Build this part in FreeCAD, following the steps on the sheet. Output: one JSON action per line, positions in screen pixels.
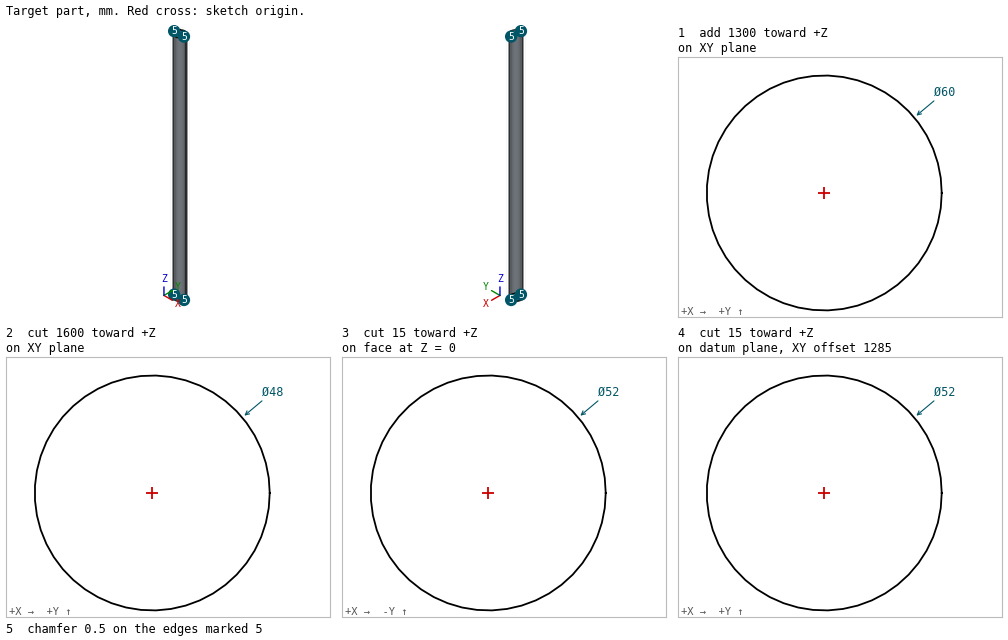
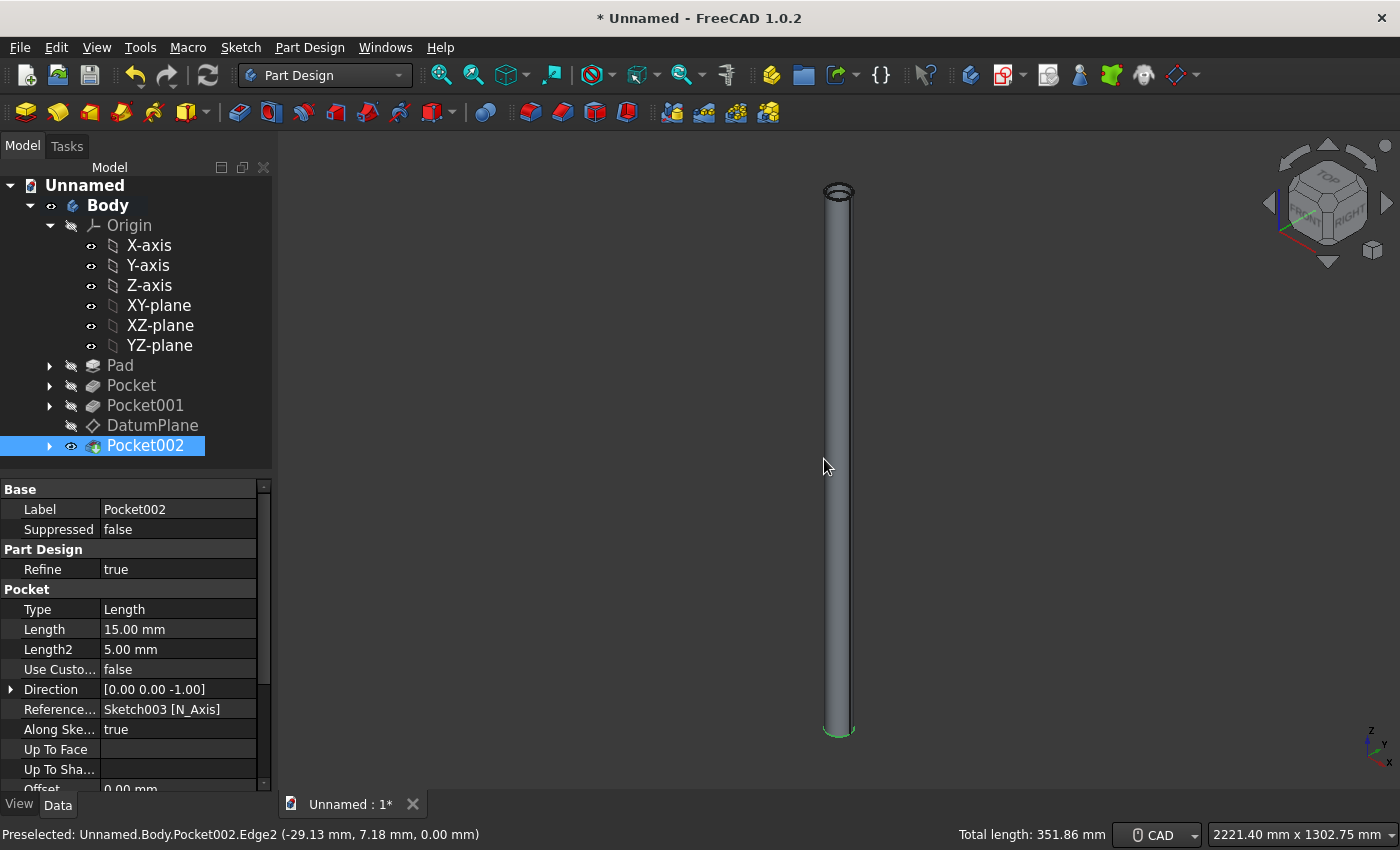
{"action": "left_click", "coordinate": [830, 186], "text": "ctrl"}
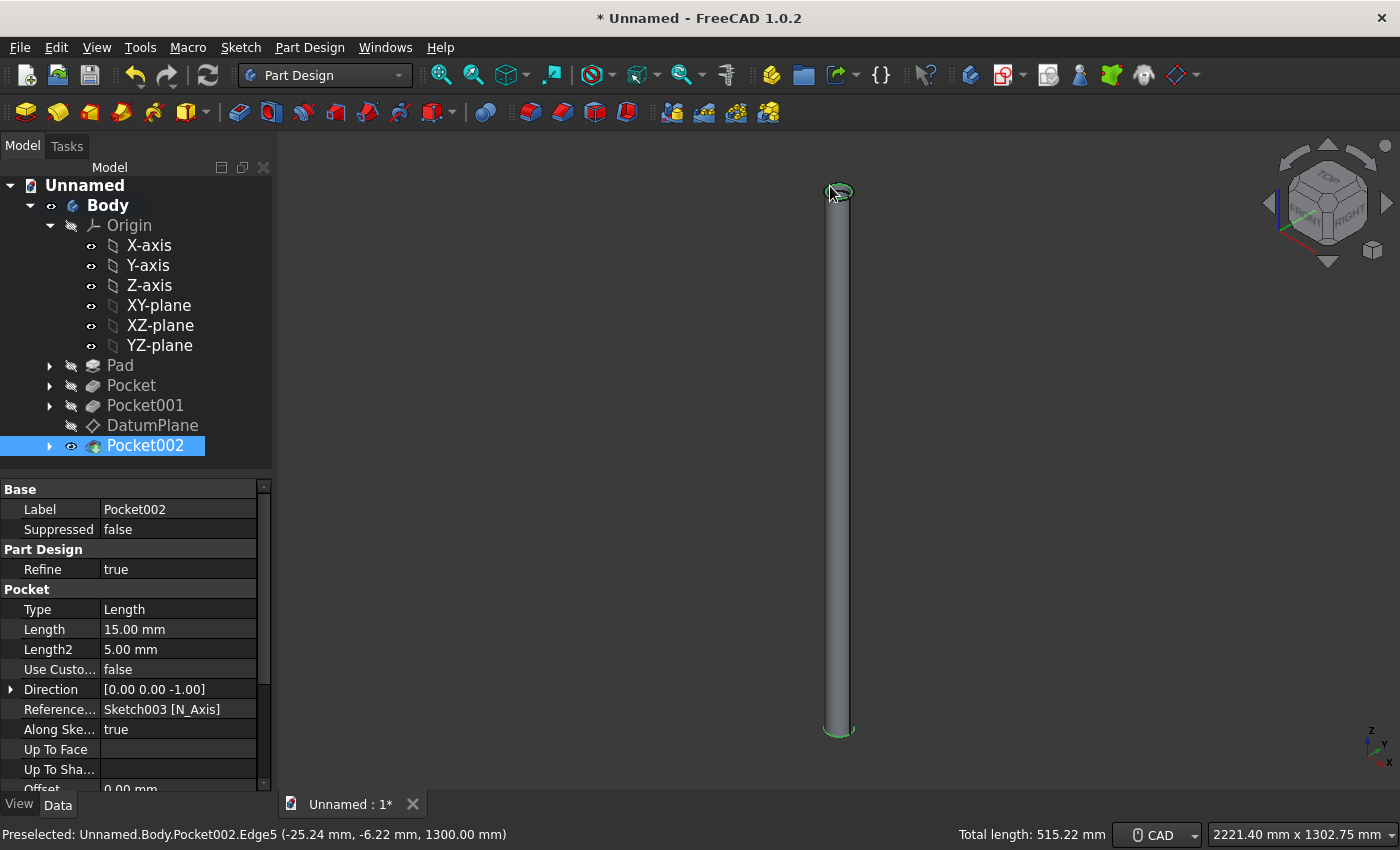
{"action": "left_click", "coordinate": [825, 195], "text": "ctrl"}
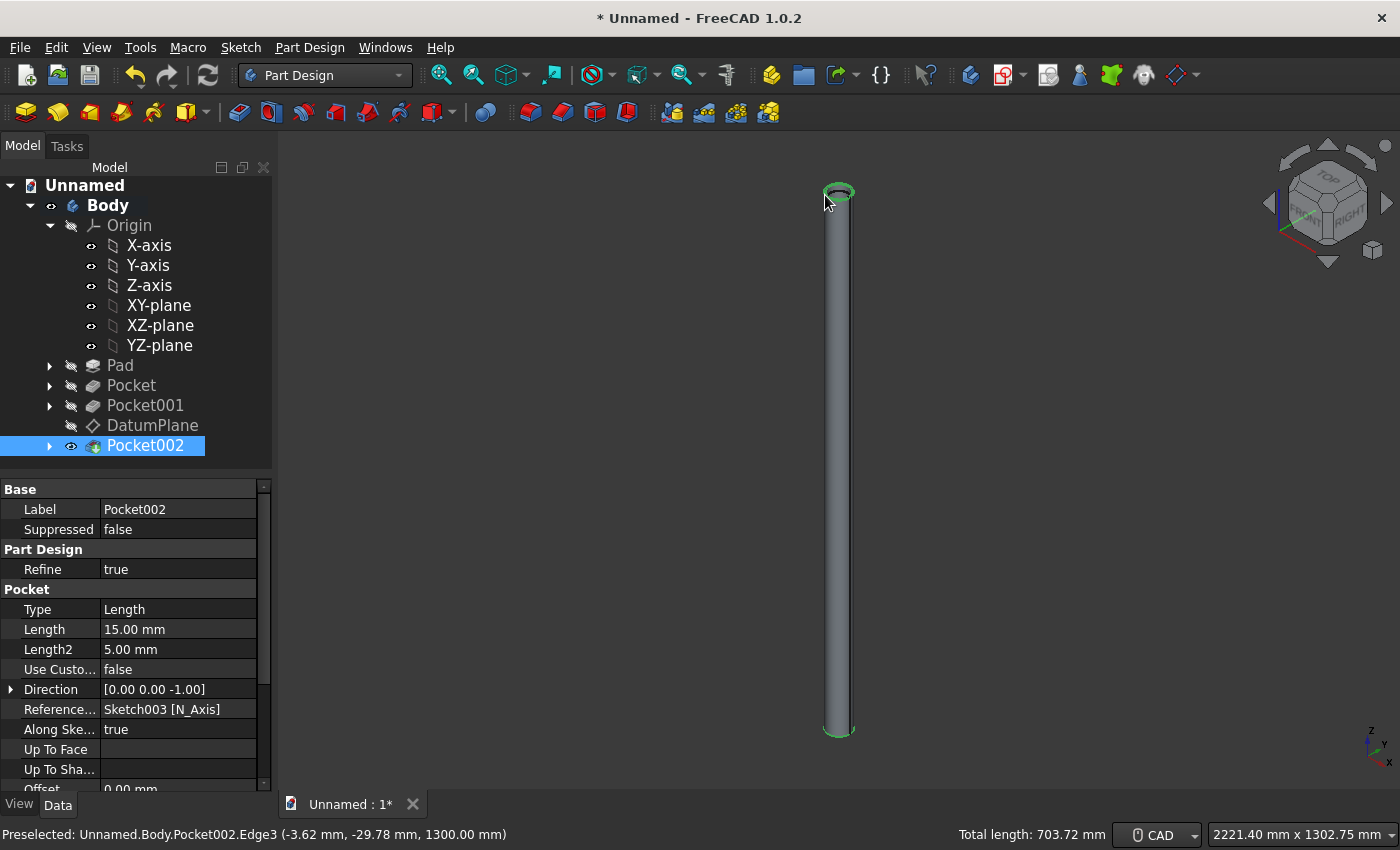
{"action": "left_click", "coordinate": [564, 112]}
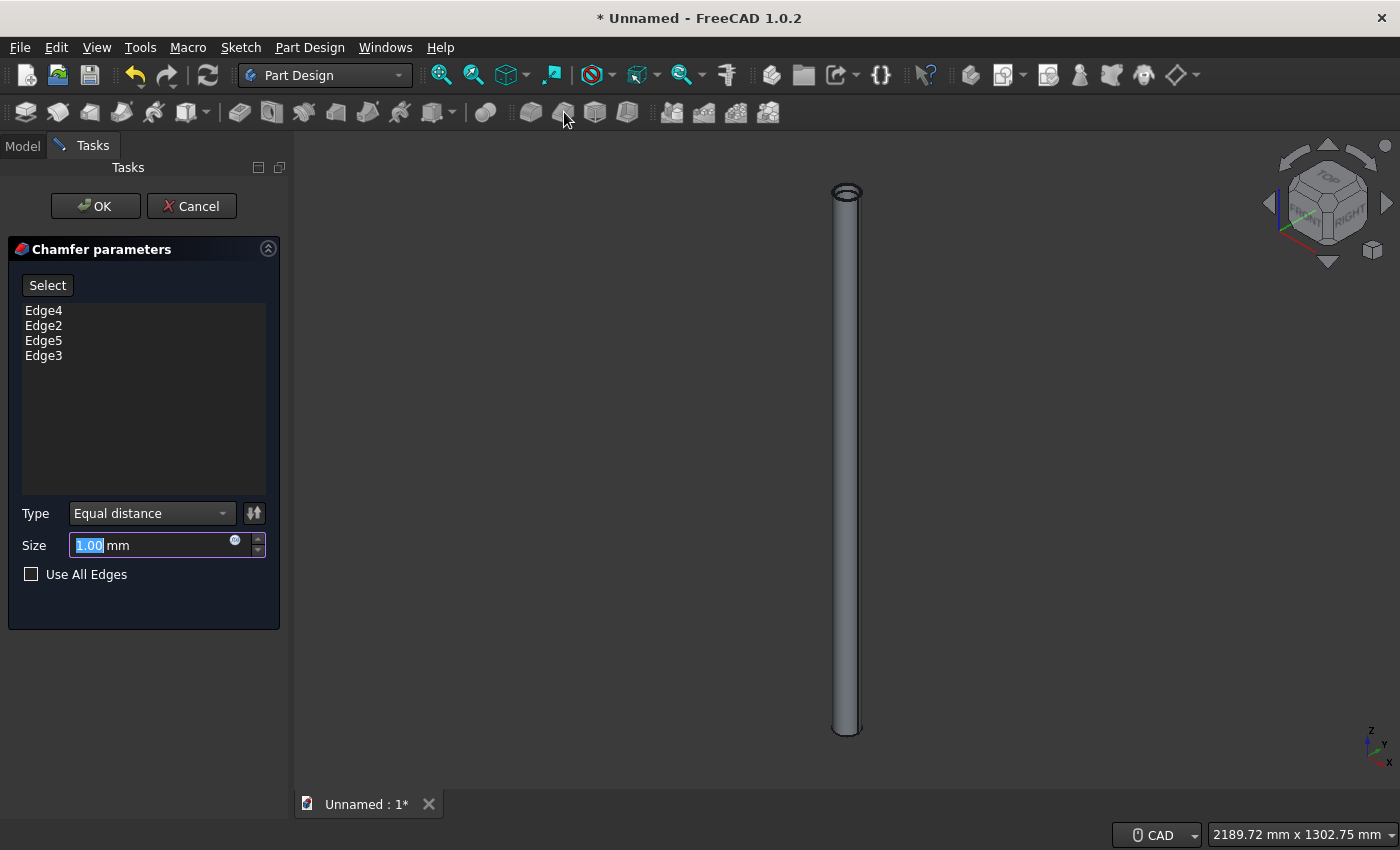
{"action": "type", "text": "0.5"}
{"action": "key", "text": "Tab"}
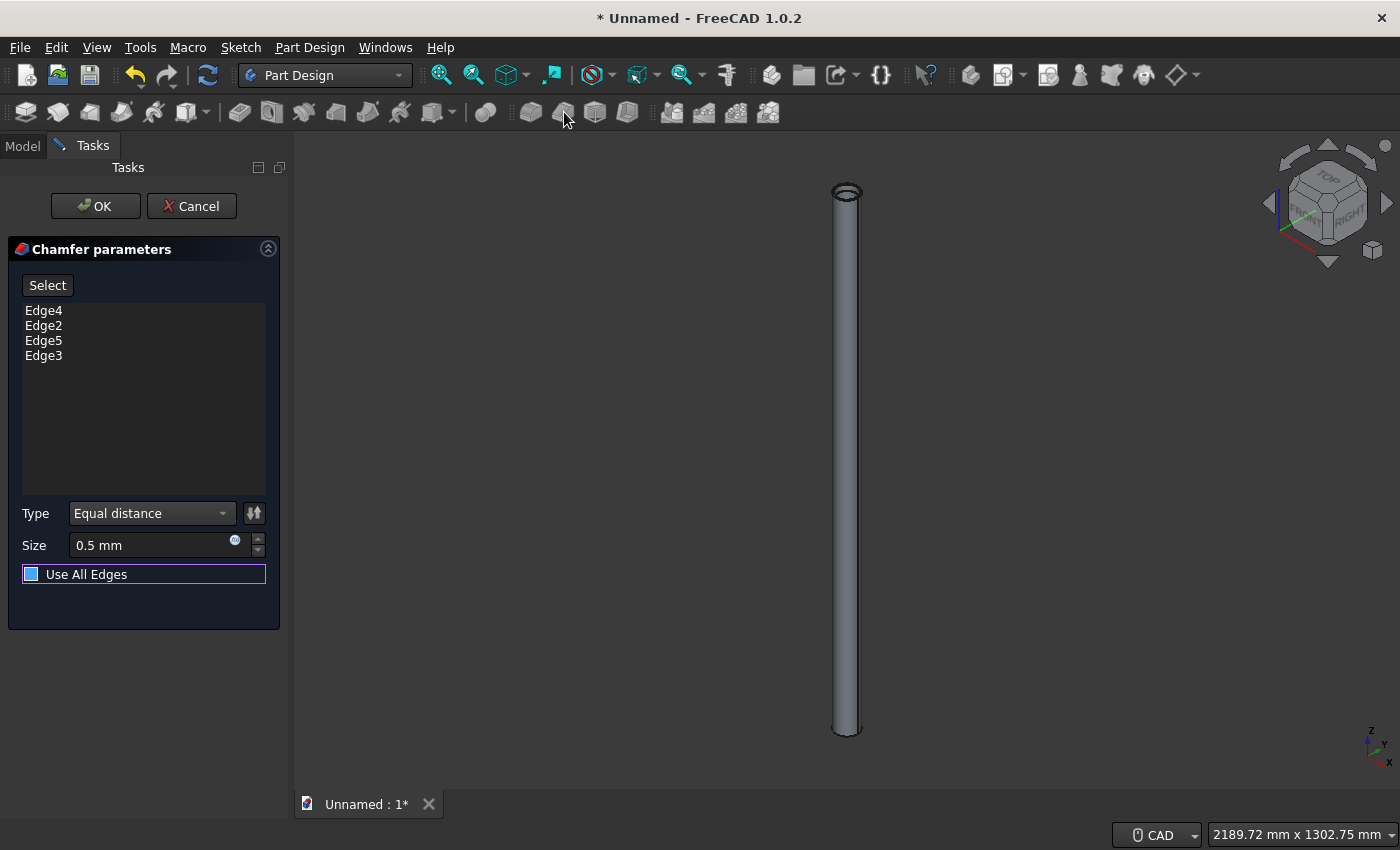
{"action": "left_click", "coordinate": [96, 206]}